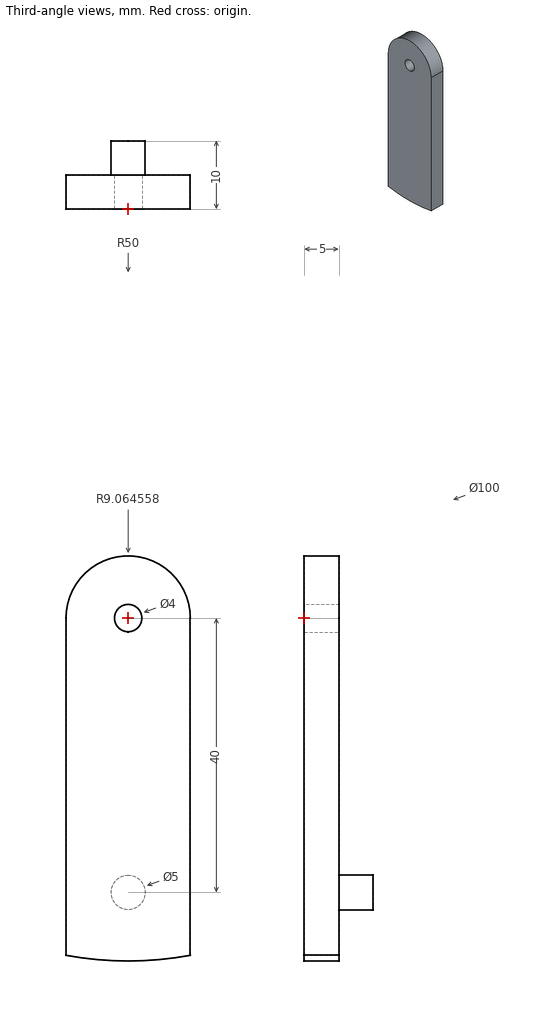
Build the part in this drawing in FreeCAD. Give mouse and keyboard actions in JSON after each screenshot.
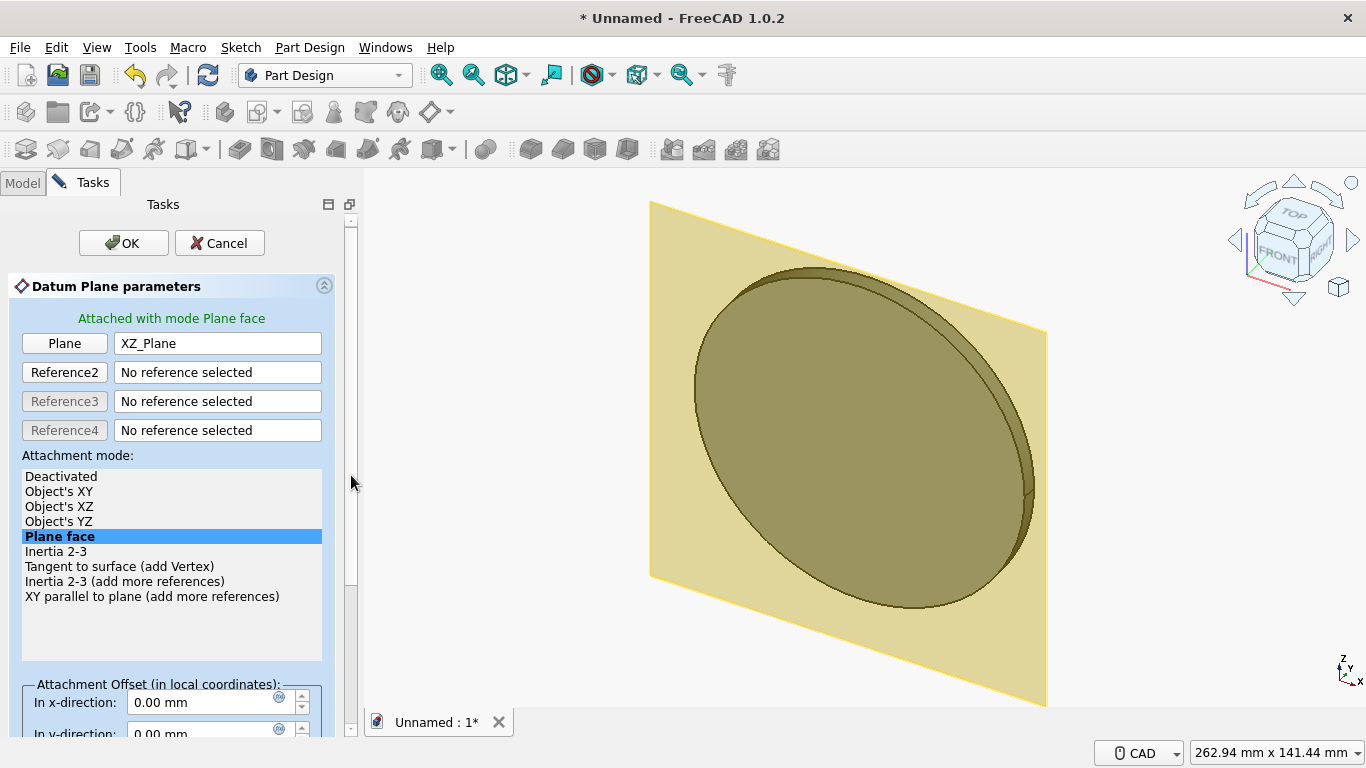
{"action": "left_click", "coordinate": [124, 243]}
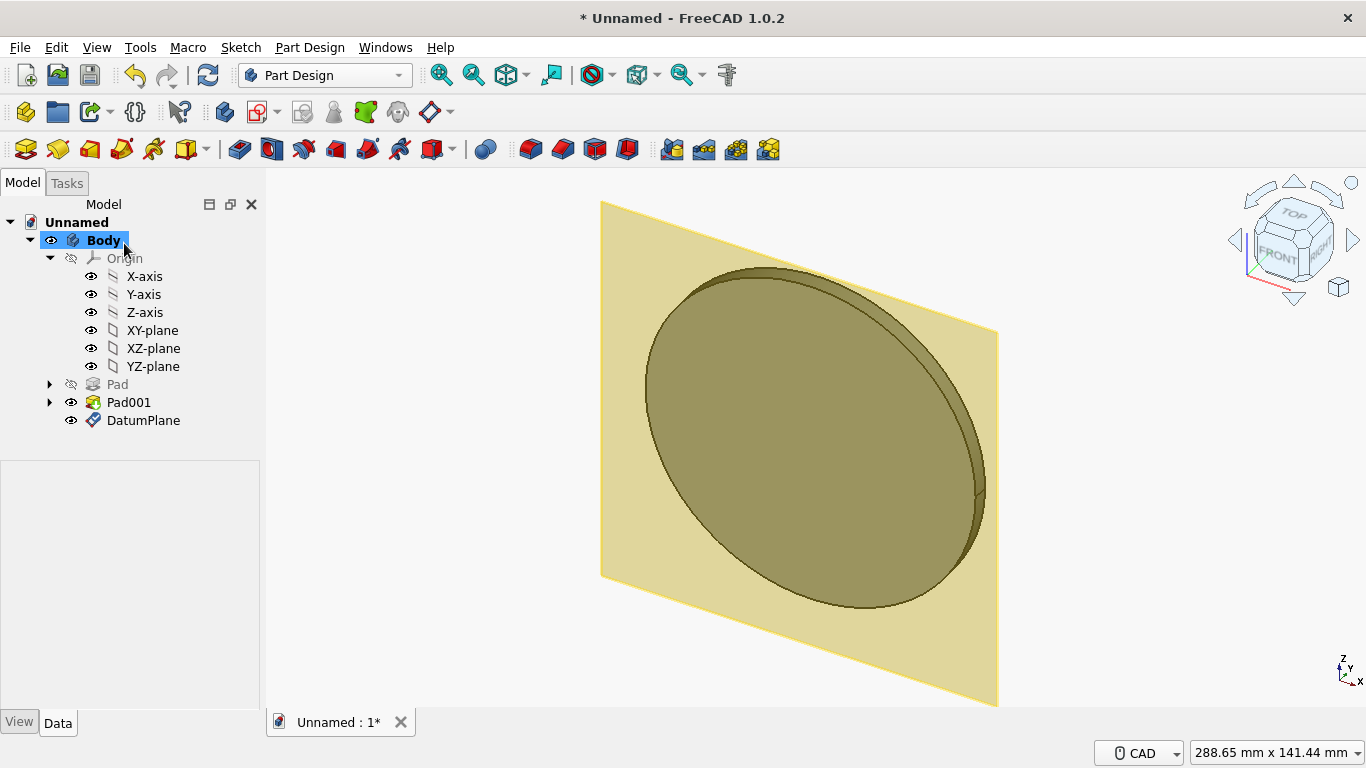
{"action": "left_click", "coordinate": [116, 420]}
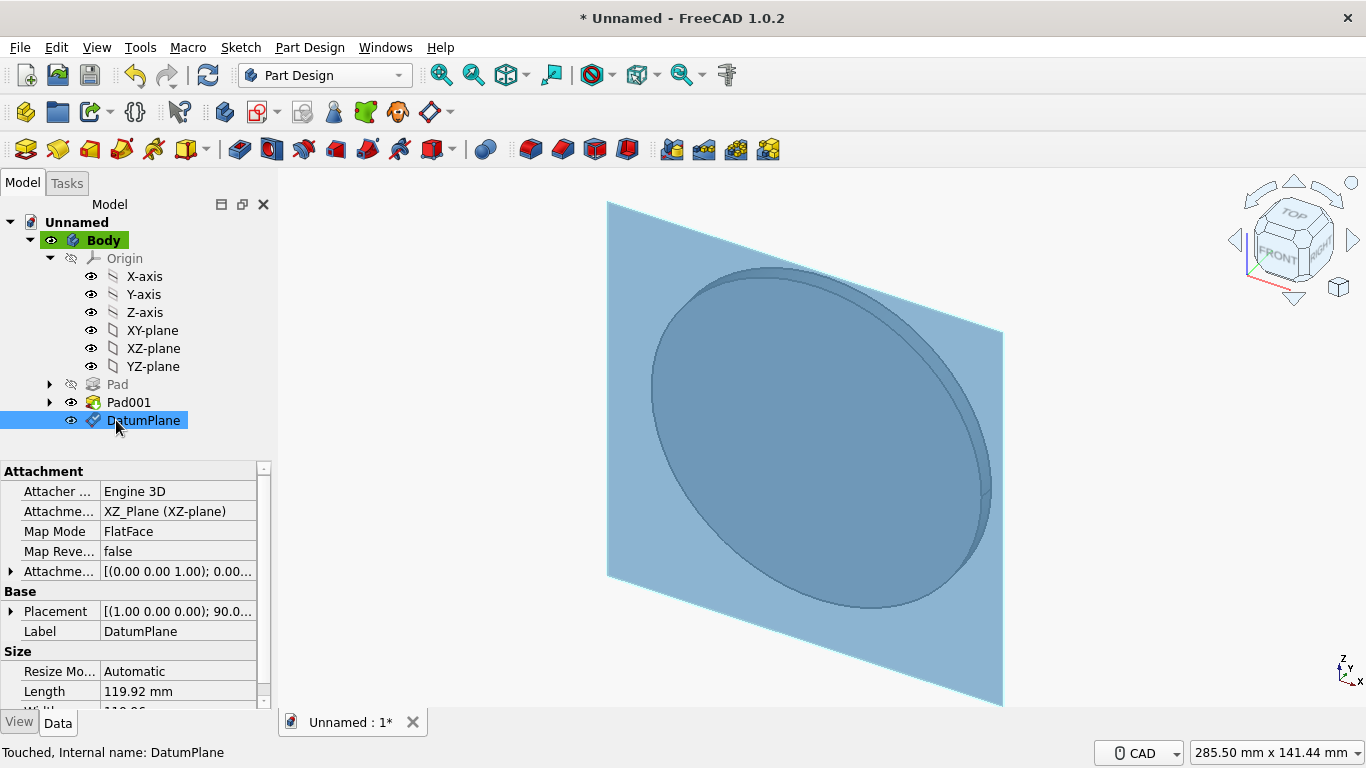
{"action": "left_click", "coordinate": [258, 112]}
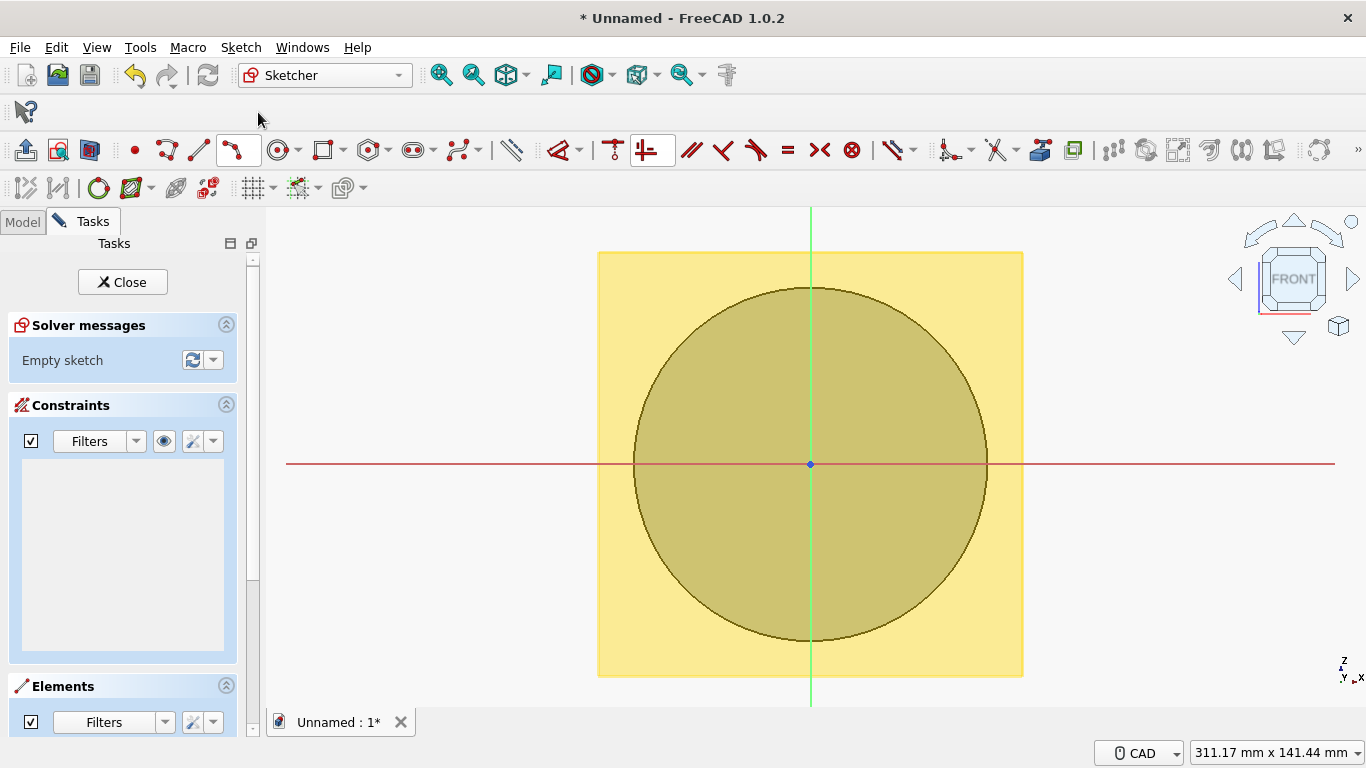
{"action": "key", "text": "g l"}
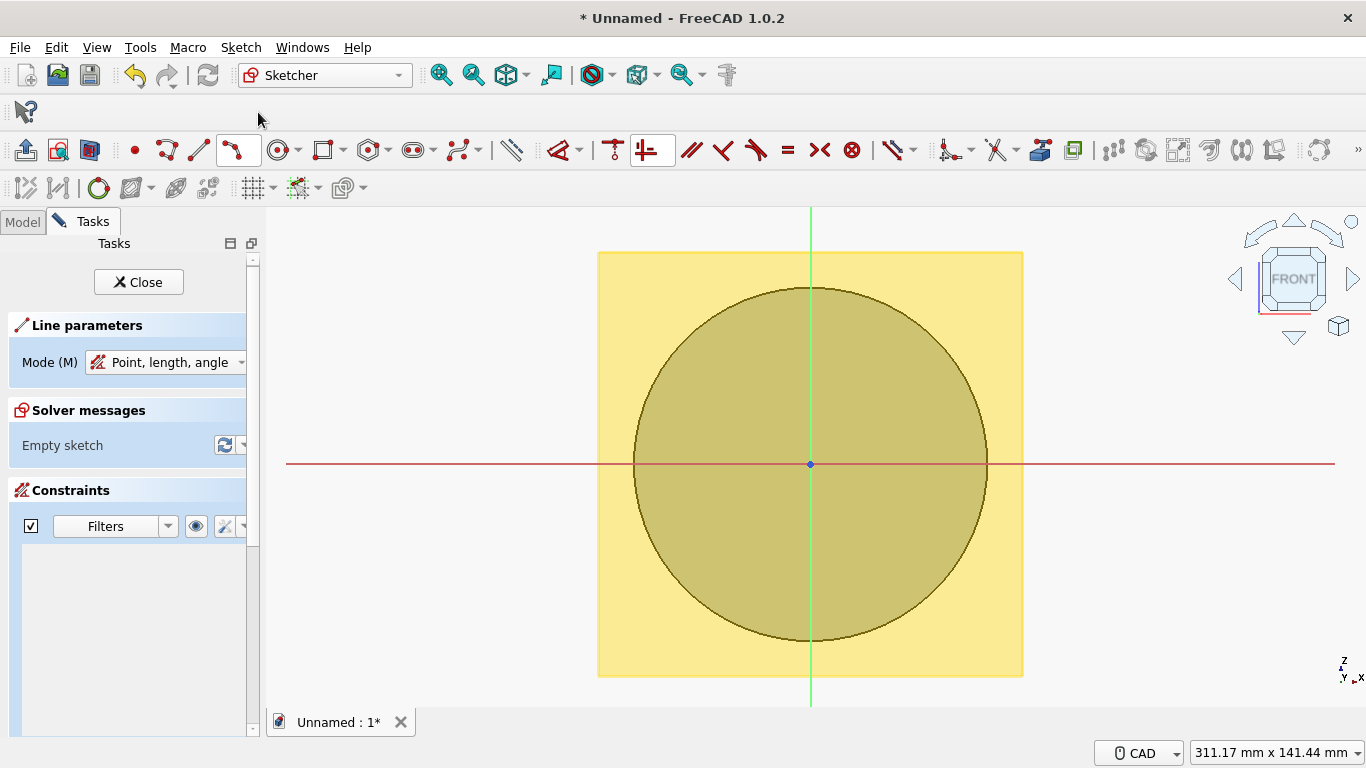
{"action": "left_click", "coordinate": [779, 464]}
{"action": "left_click", "coordinate": [779, 638]}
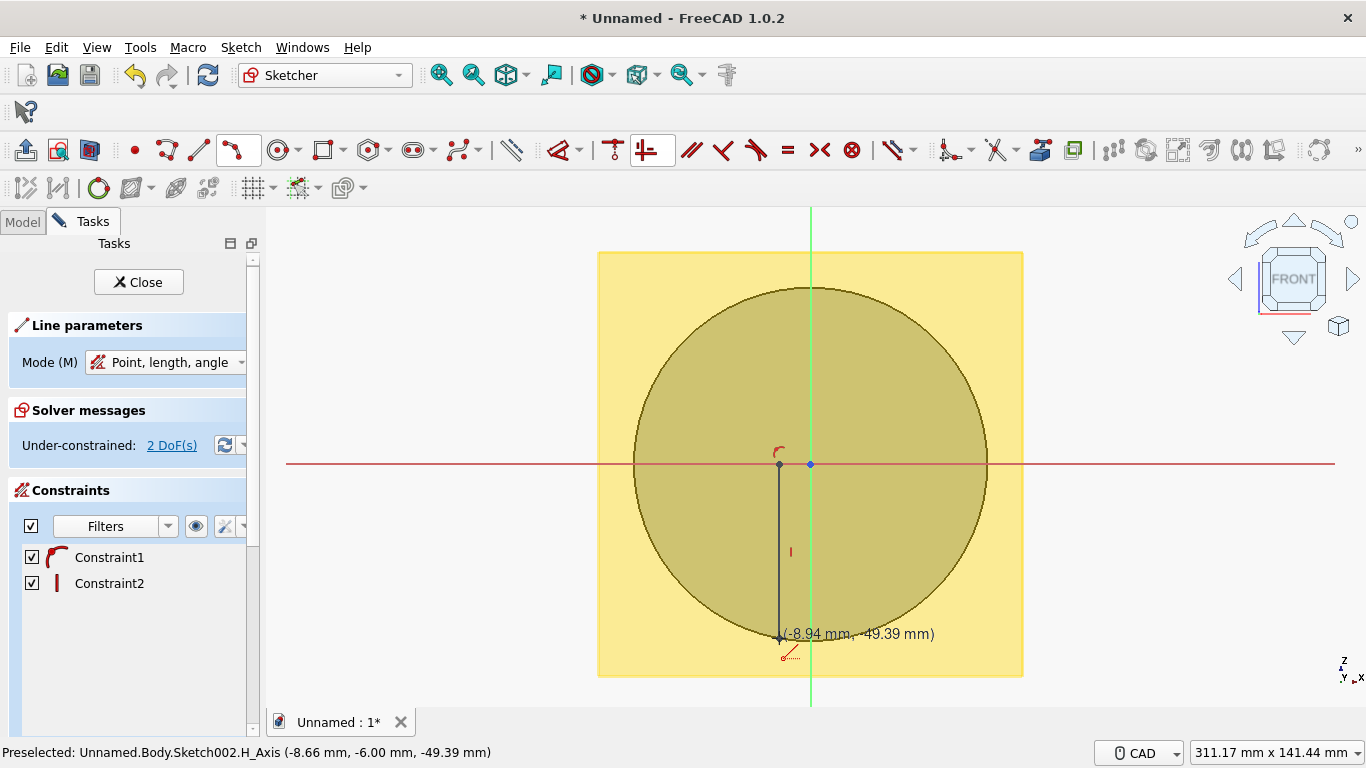
{"action": "left_click", "coordinate": [843, 638]}
{"action": "left_click", "coordinate": [843, 464]}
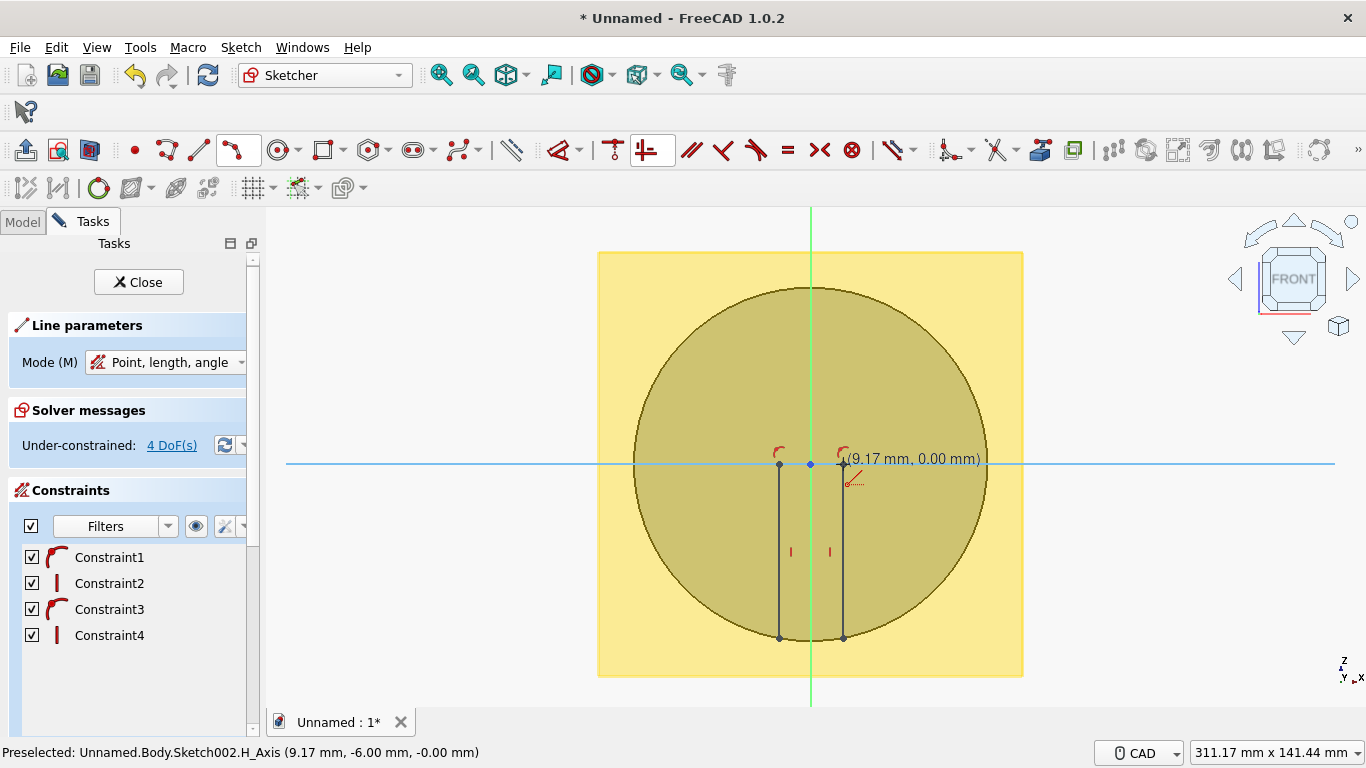
{"action": "left_click", "coordinate": [232, 150]}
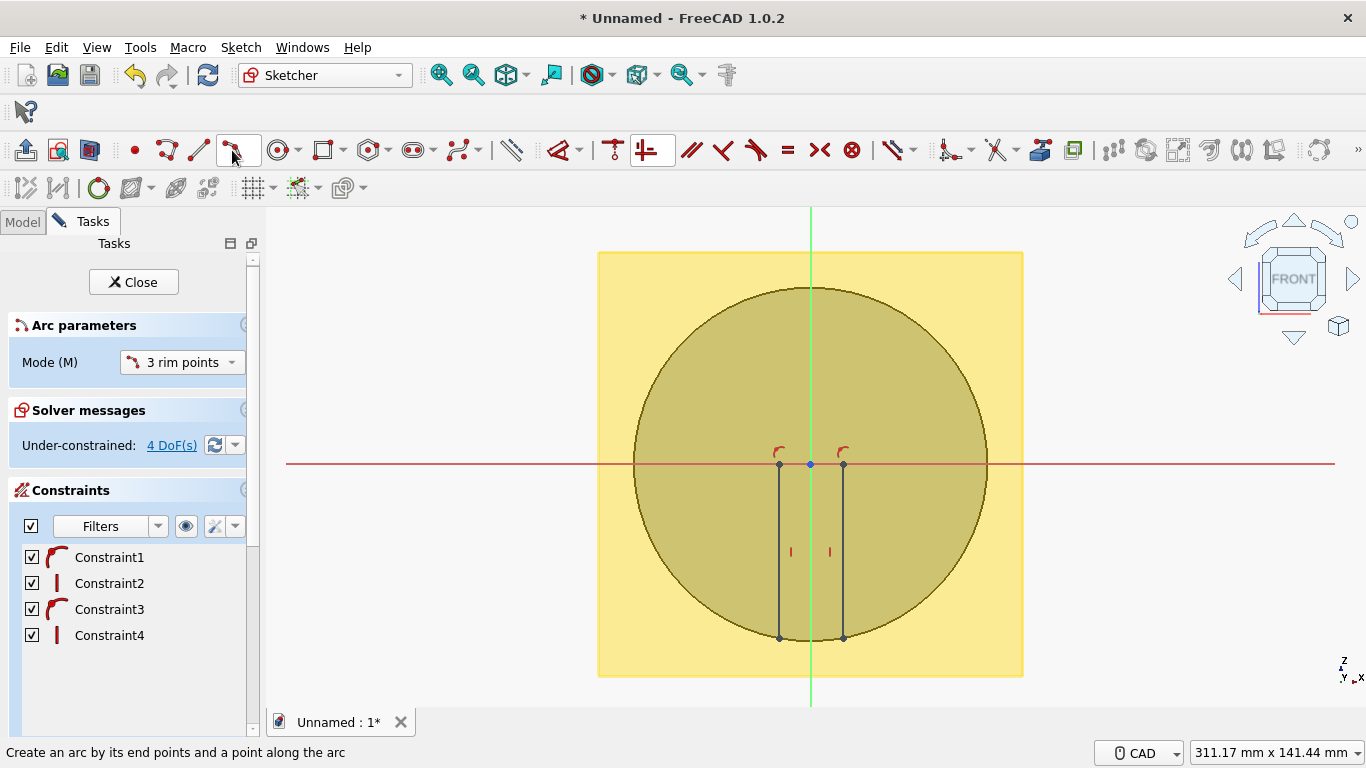
{"action": "left_click", "coordinate": [779, 639]}
{"action": "left_click", "coordinate": [843, 639]}
{"action": "left_click", "coordinate": [909, 318]}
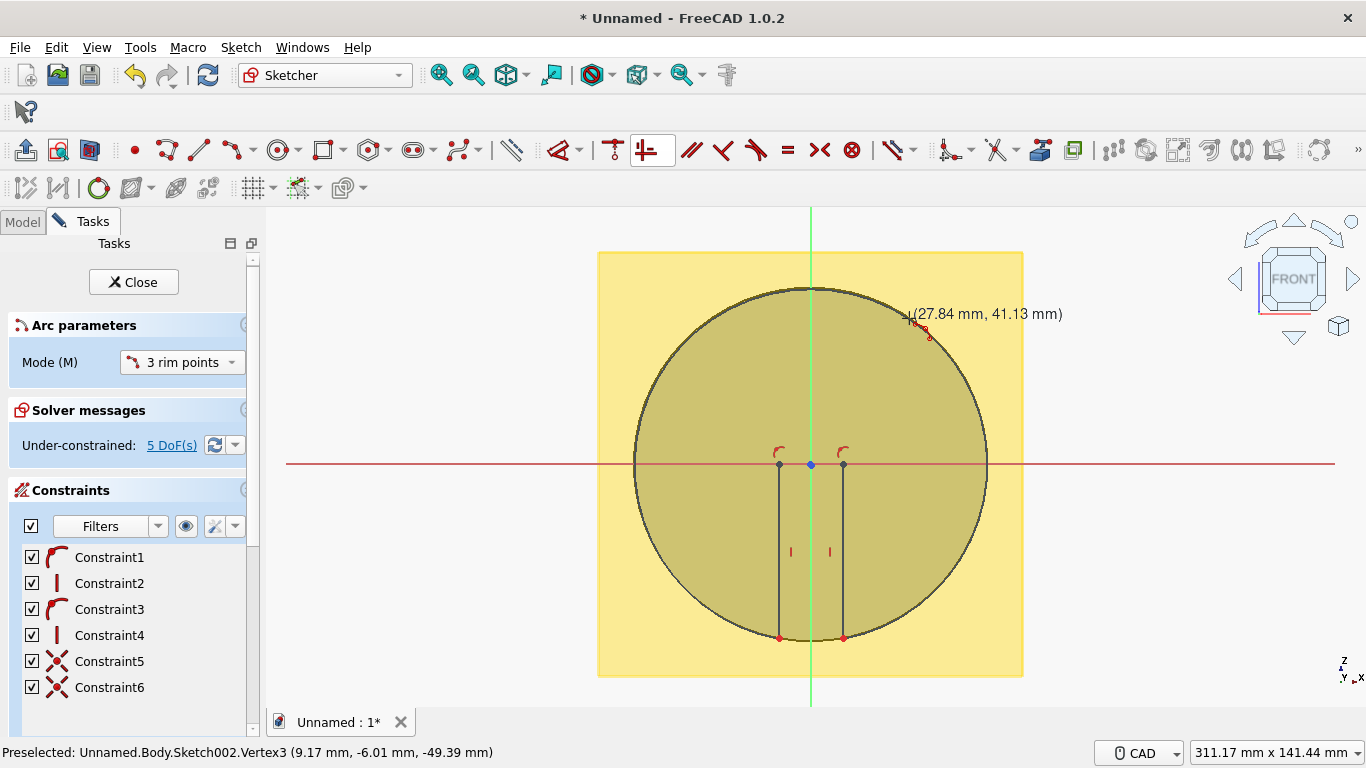
{"action": "left_click", "coordinate": [843, 464]}
{"action": "left_click", "coordinate": [779, 464]}
{"action": "left_click", "coordinate": [829, 438]}
{"action": "key", "text": "Escape"}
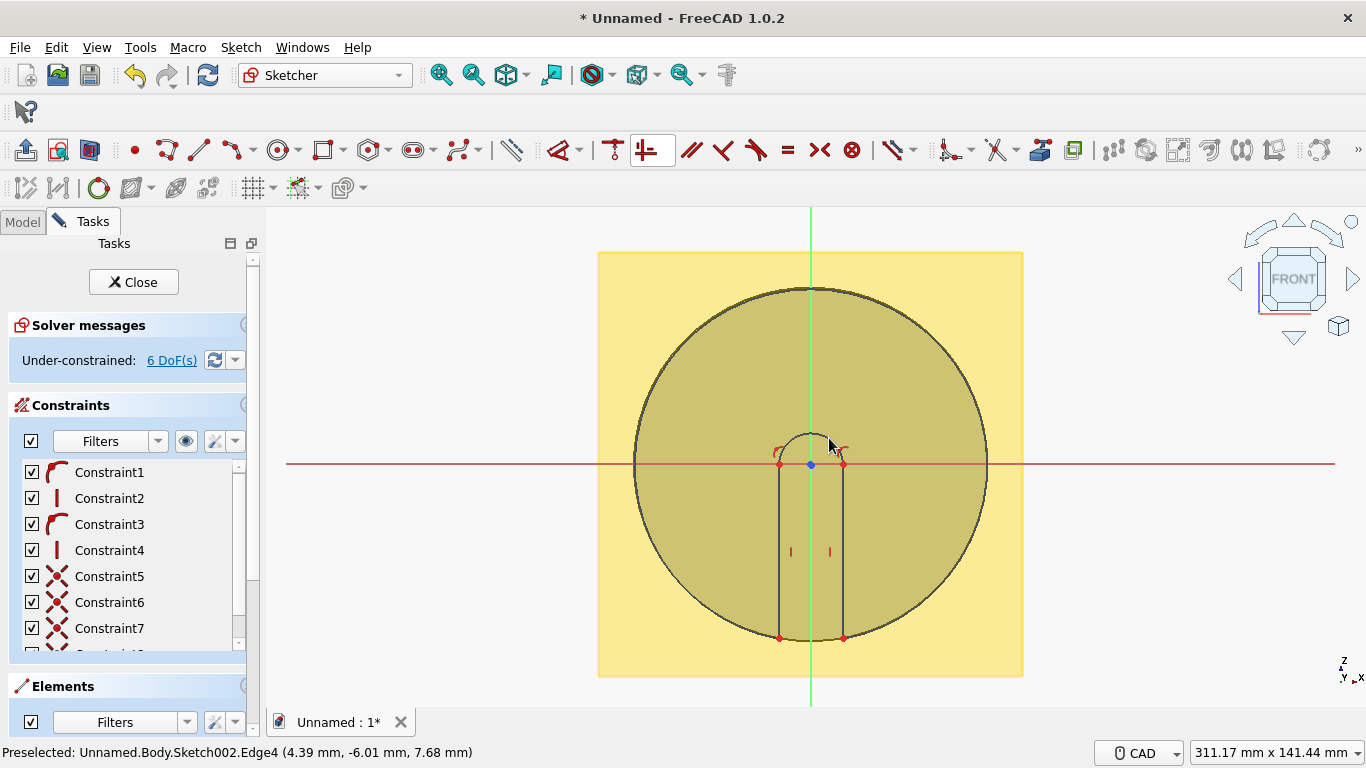
{"action": "left_click", "coordinate": [779, 517]}